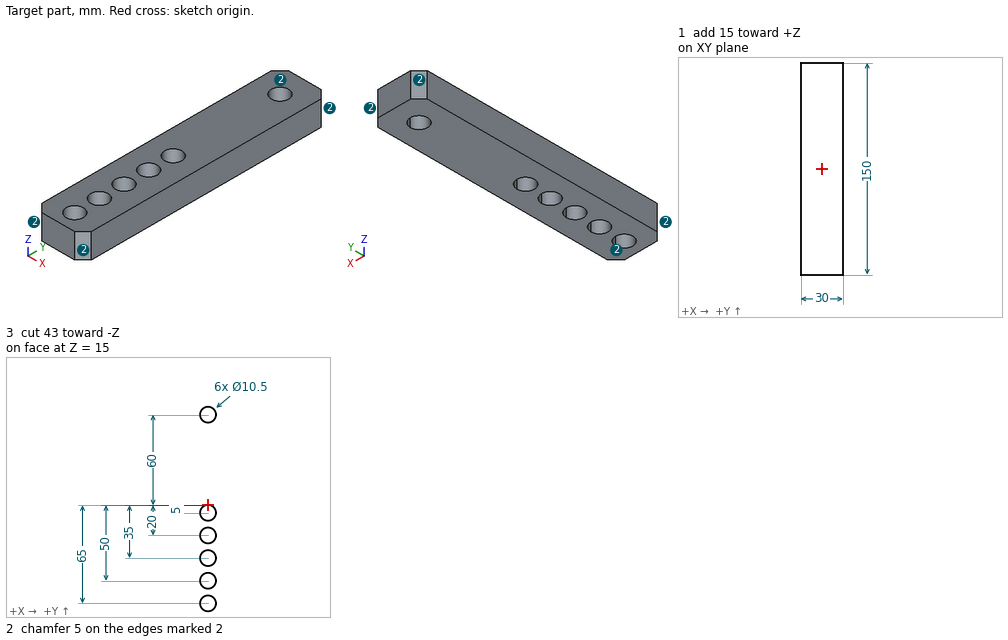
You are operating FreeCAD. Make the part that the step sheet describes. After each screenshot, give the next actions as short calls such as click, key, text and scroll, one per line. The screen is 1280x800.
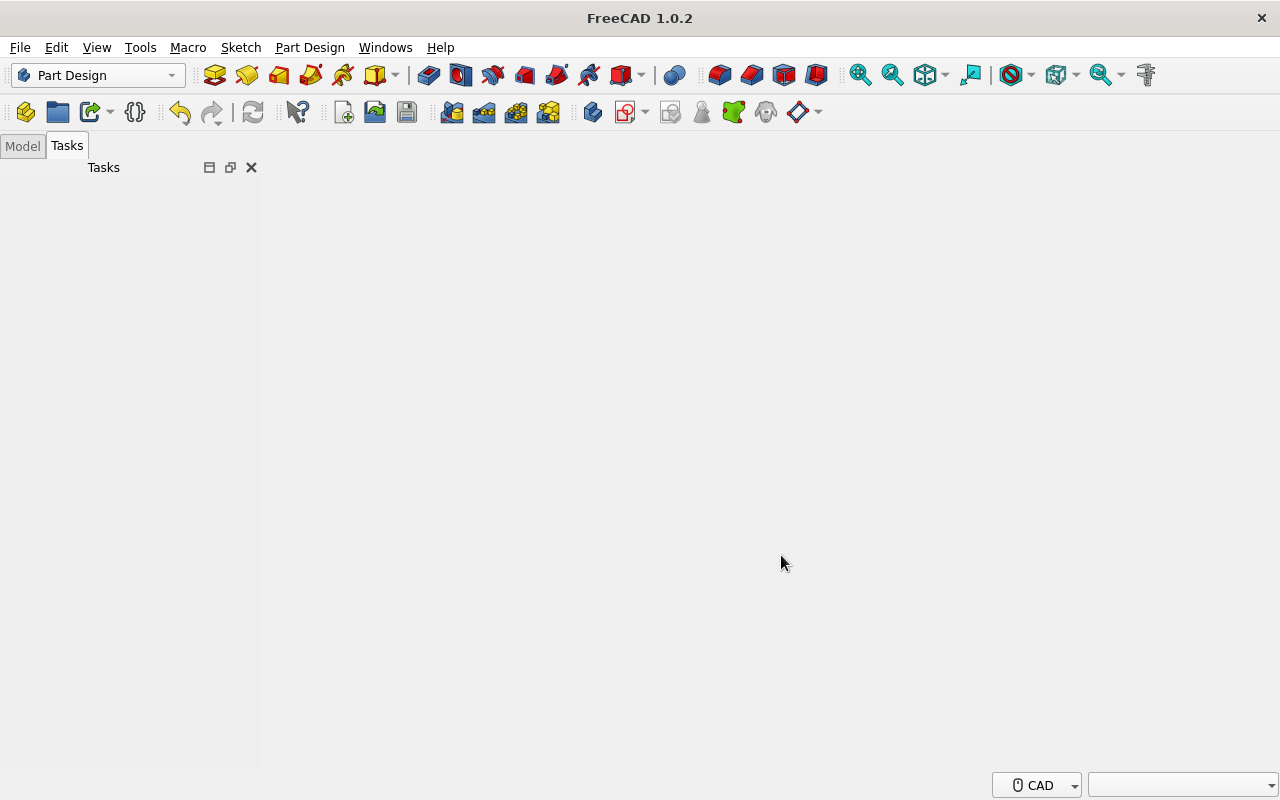
click(344, 112)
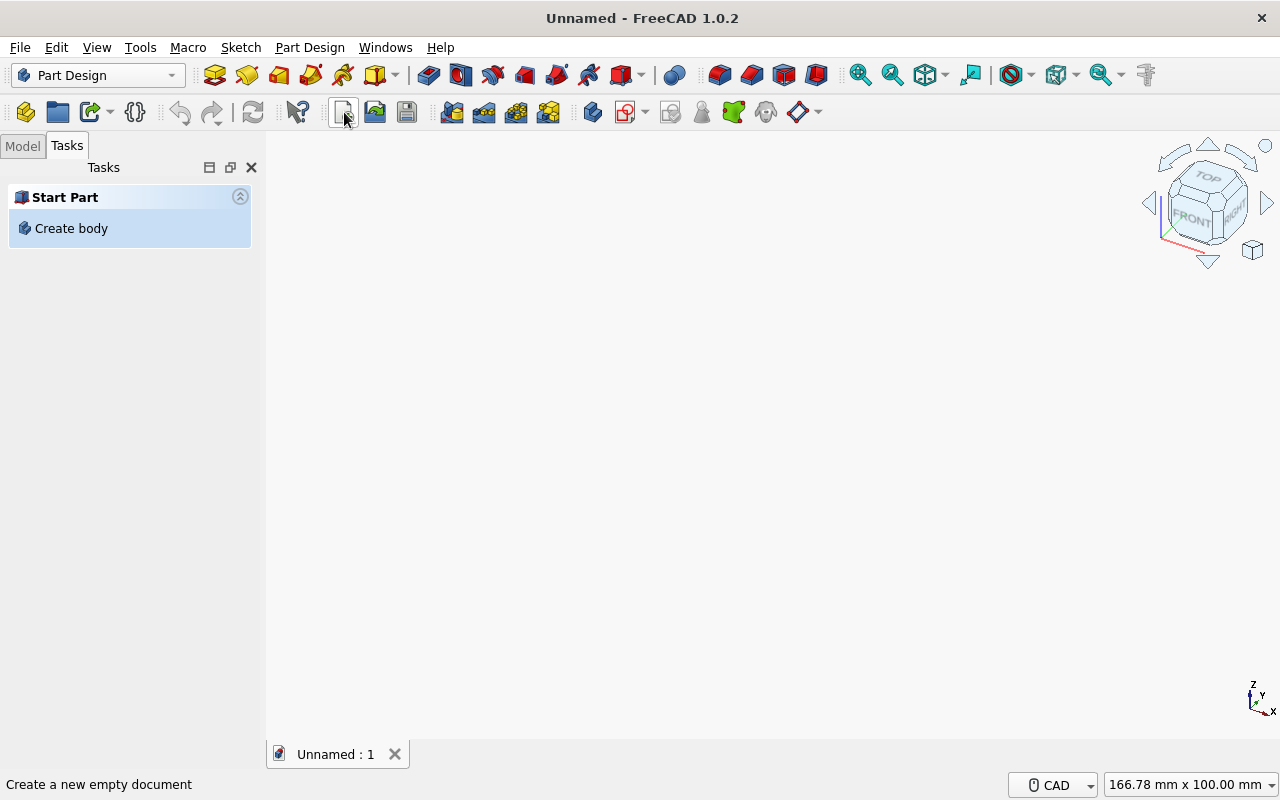
click(626, 112)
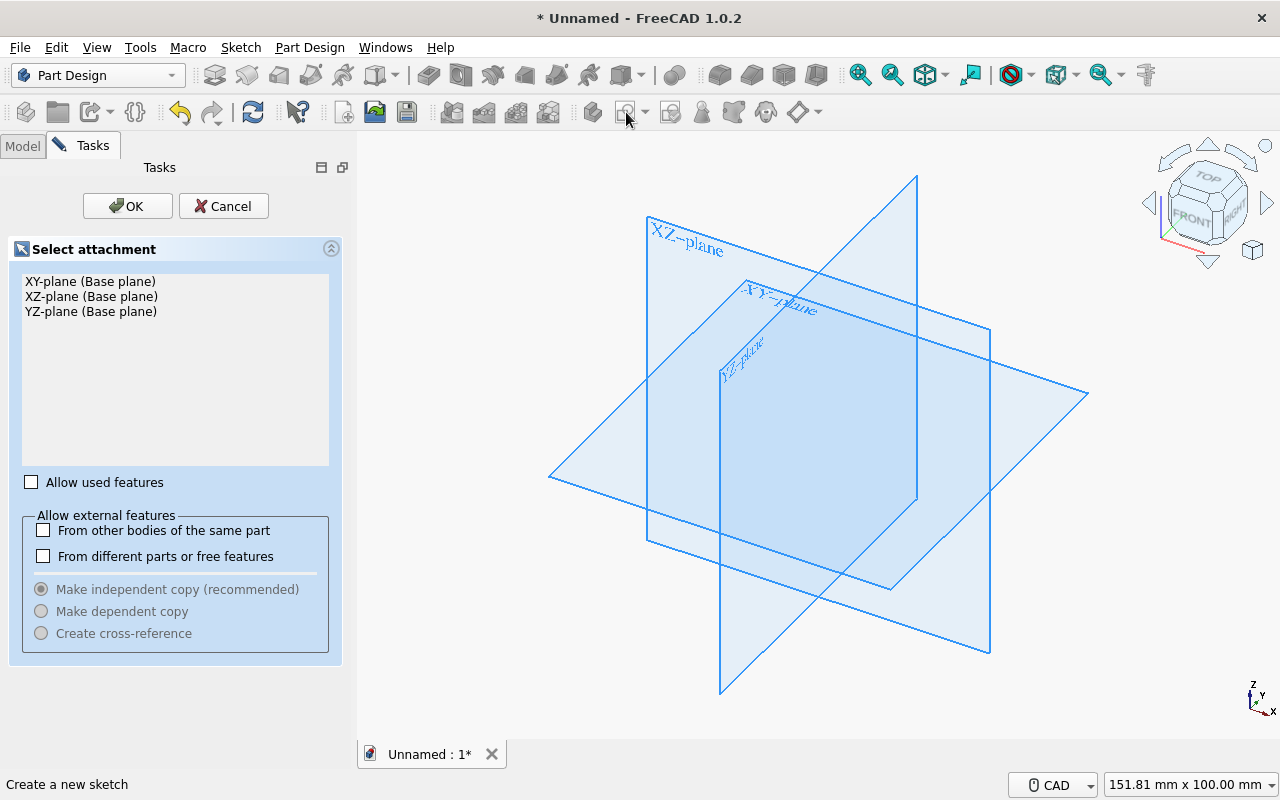
click(82, 282)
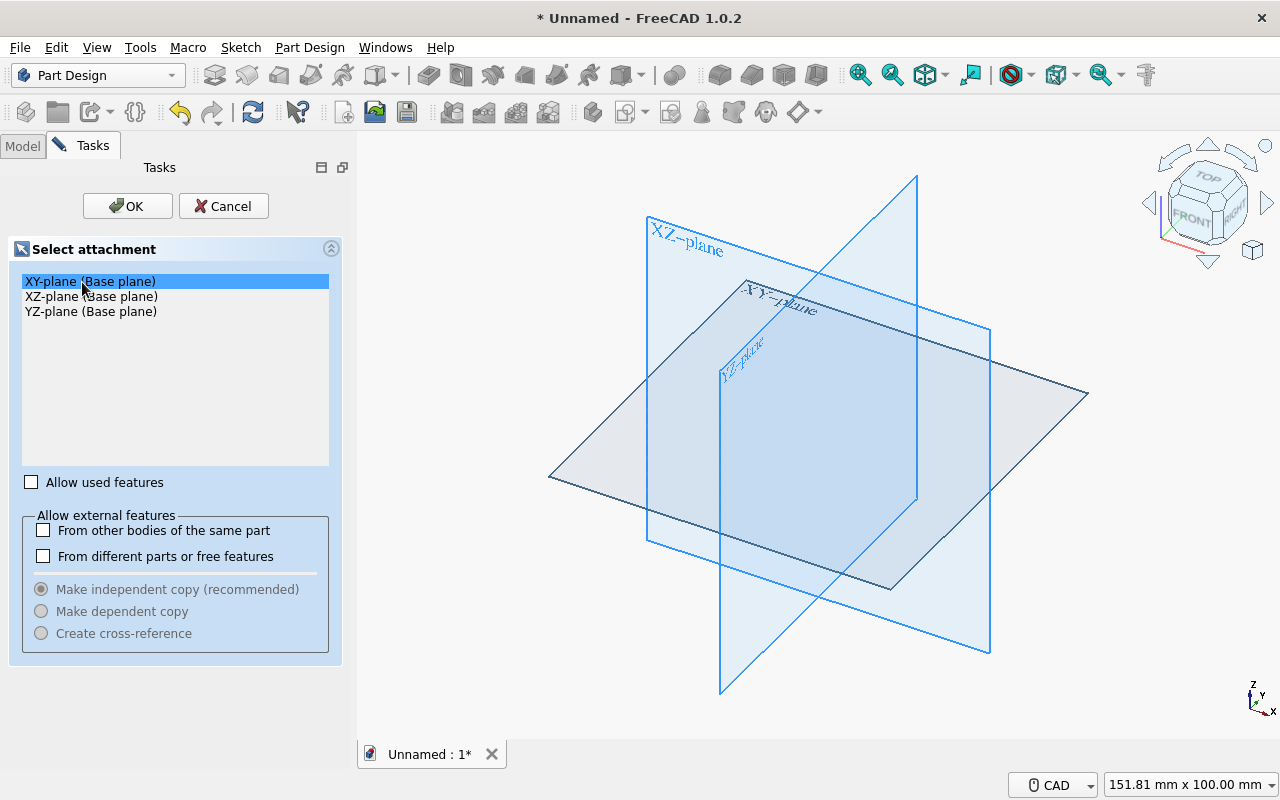
click(128, 206)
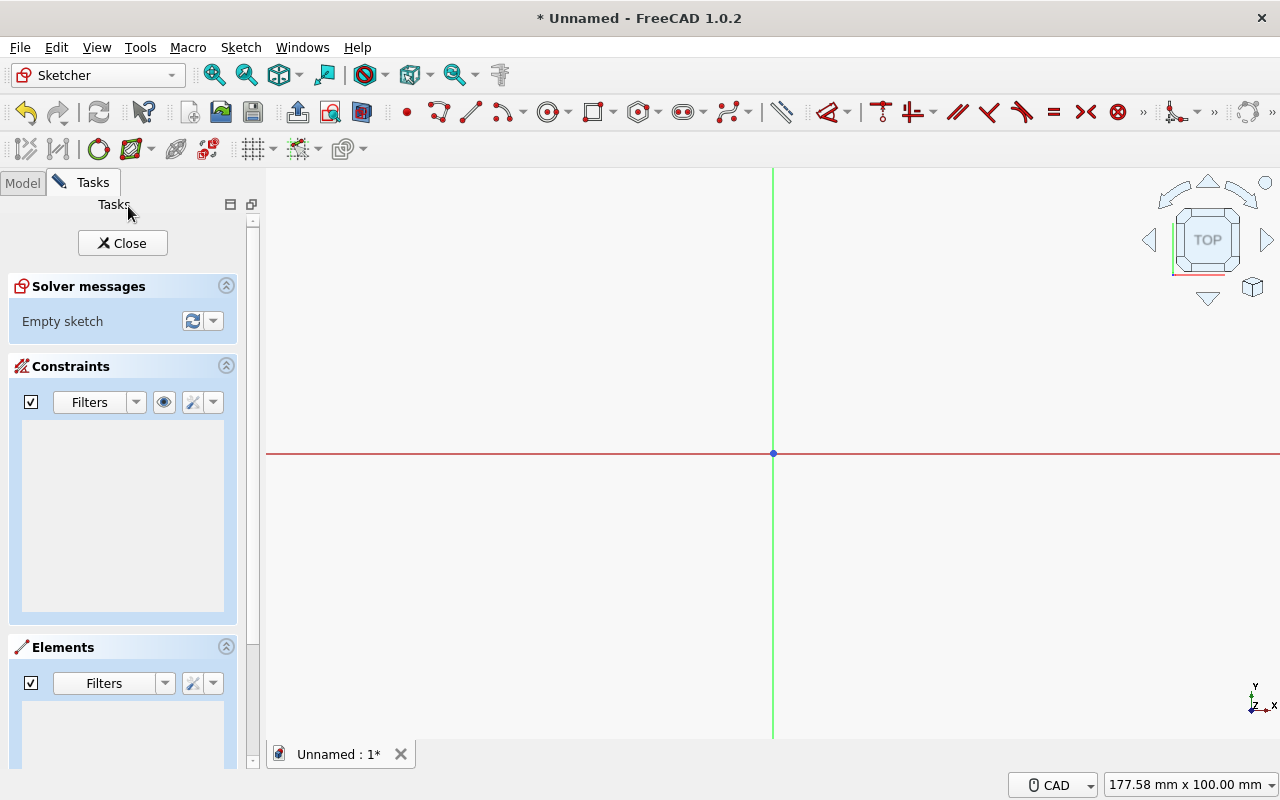
scroll(649, 454, down, 4)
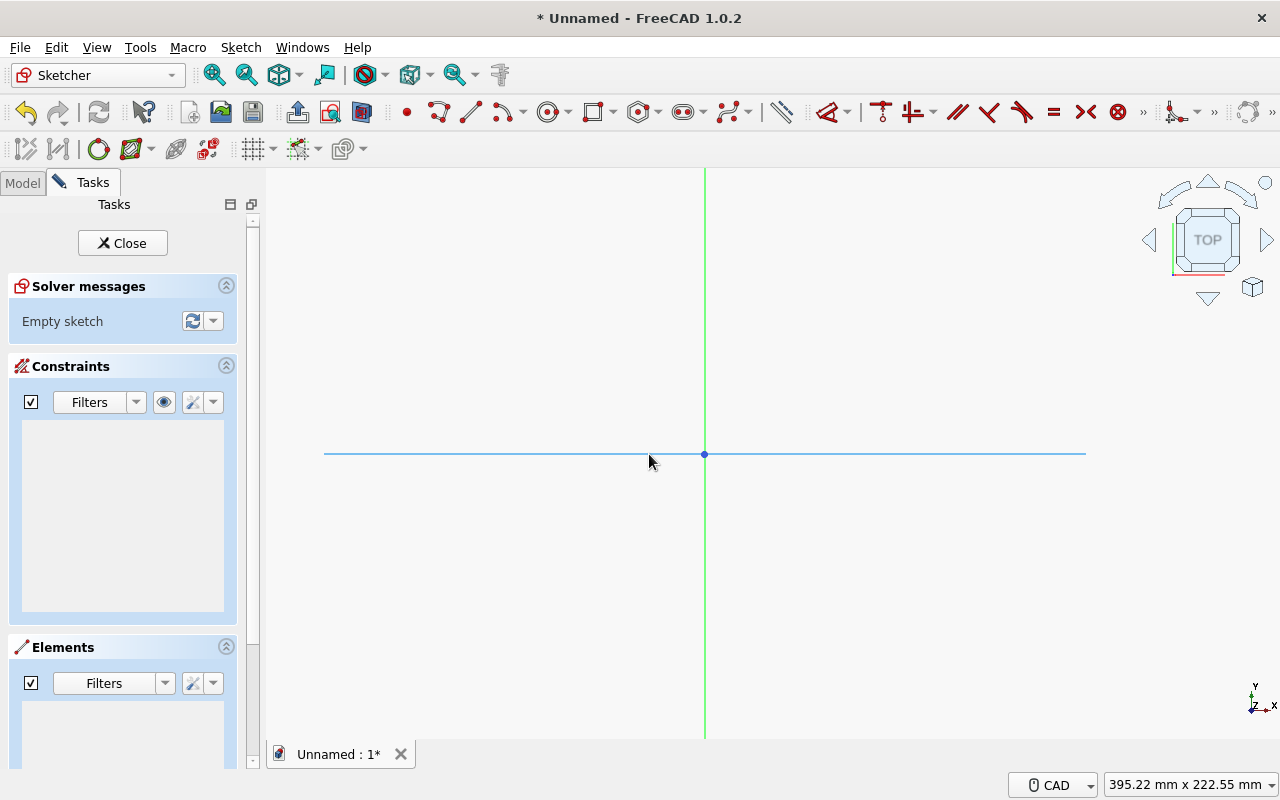
click(616, 112)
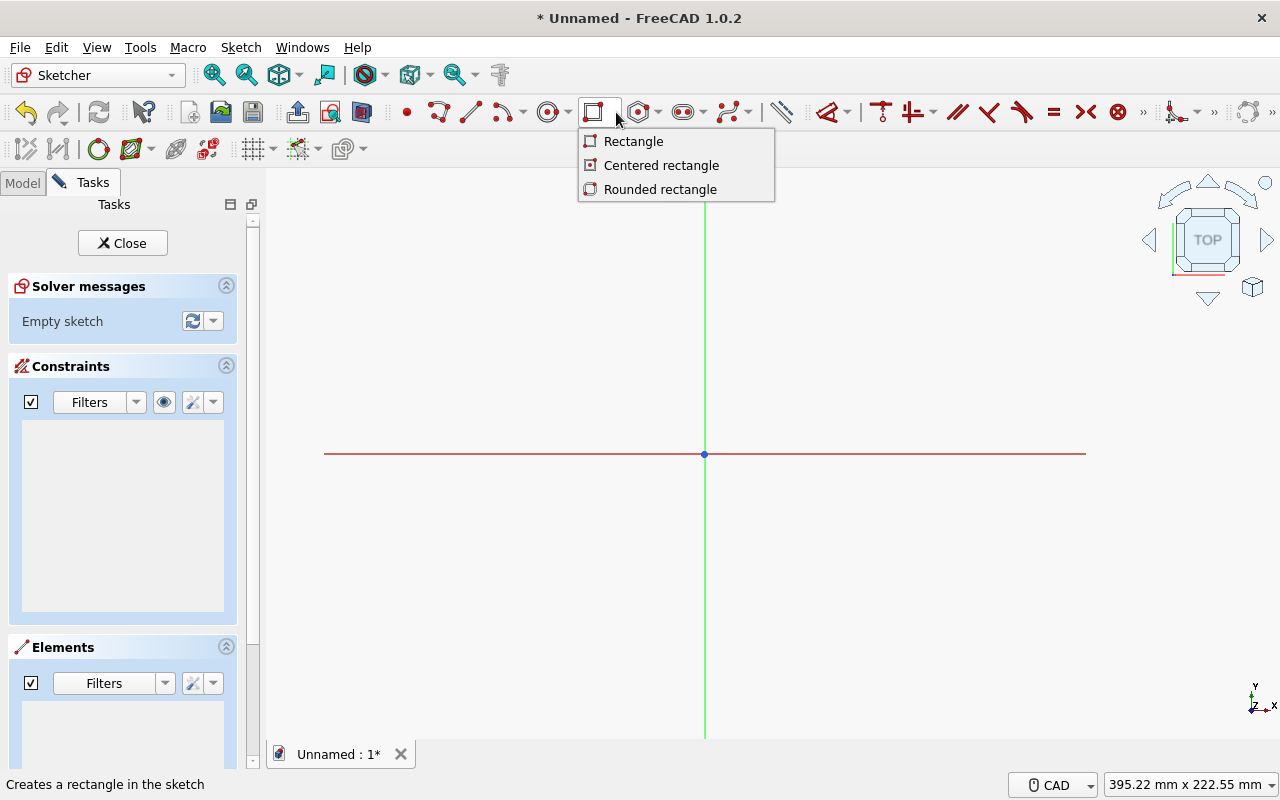
click(676, 165)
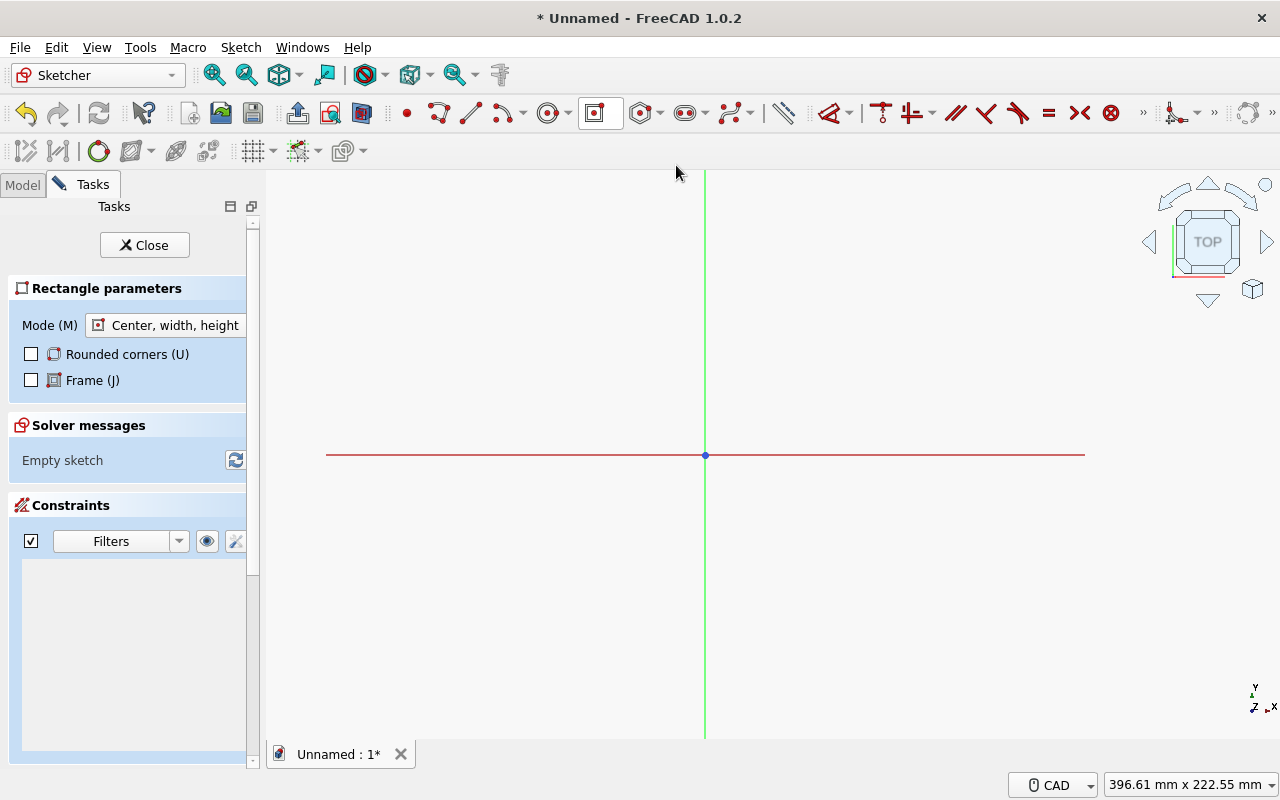
click(705, 455)
click(744, 263)
key(Escape)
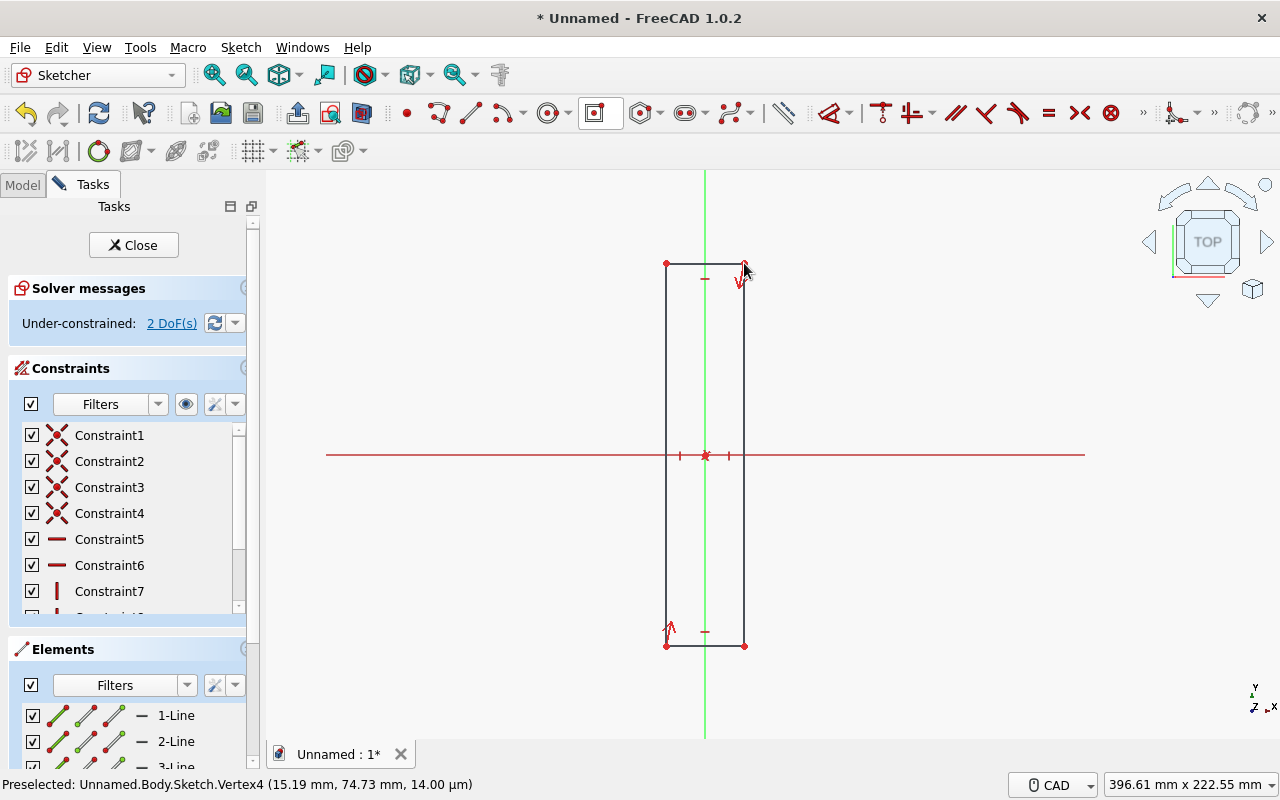
click(830, 114)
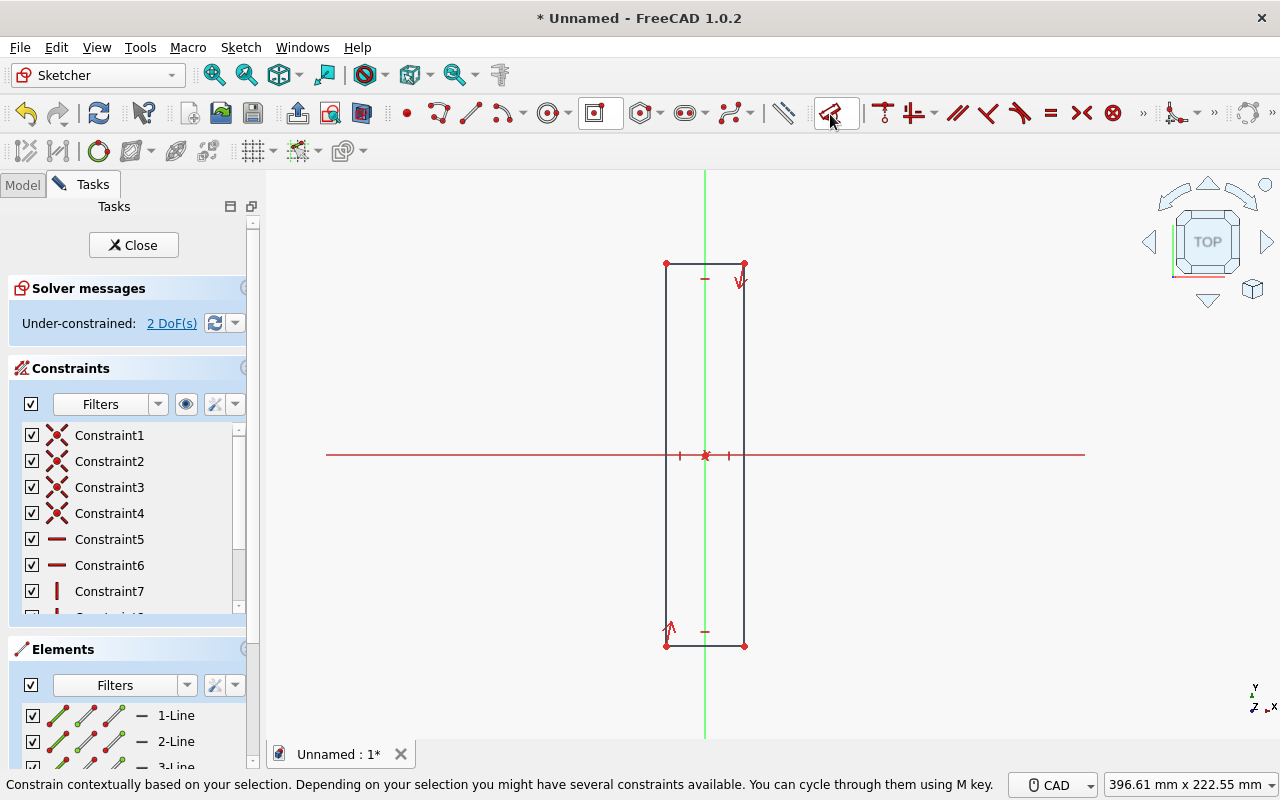
click(690, 646)
click(687, 680)